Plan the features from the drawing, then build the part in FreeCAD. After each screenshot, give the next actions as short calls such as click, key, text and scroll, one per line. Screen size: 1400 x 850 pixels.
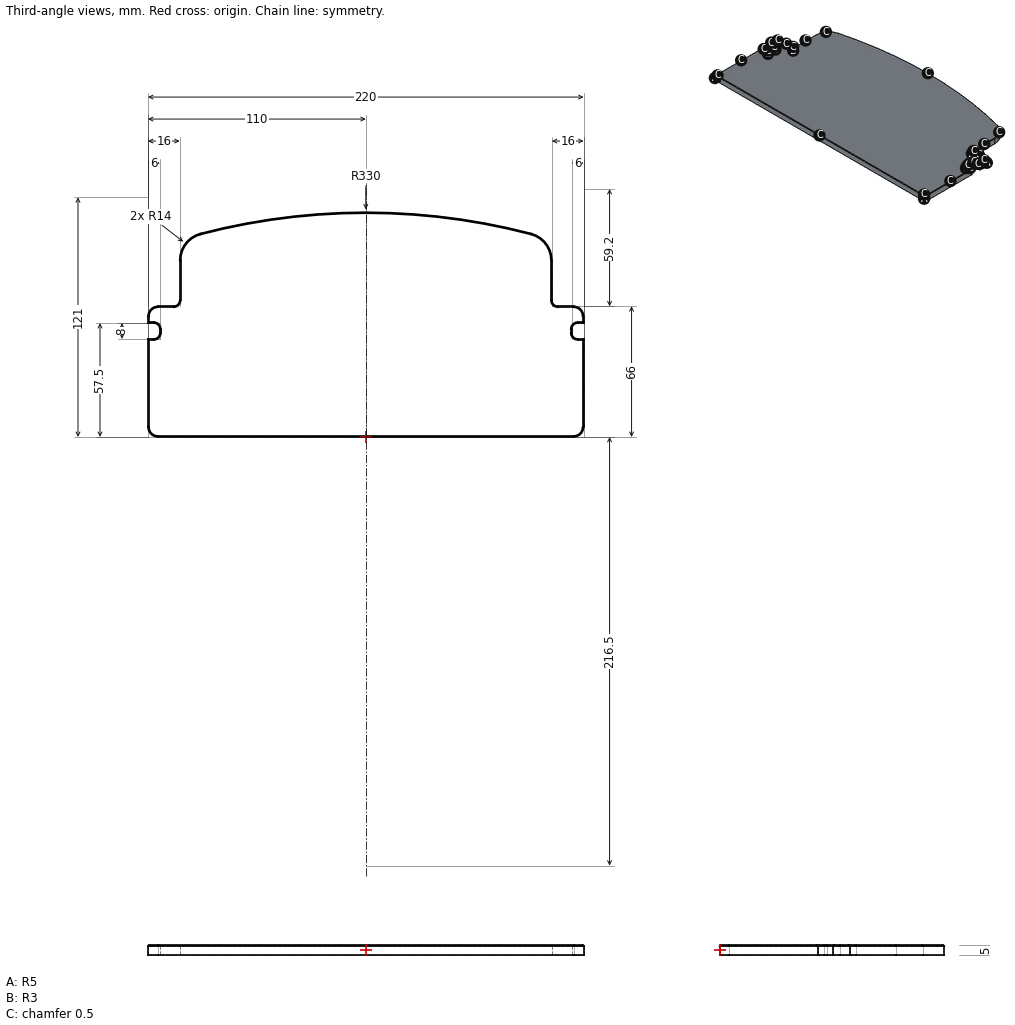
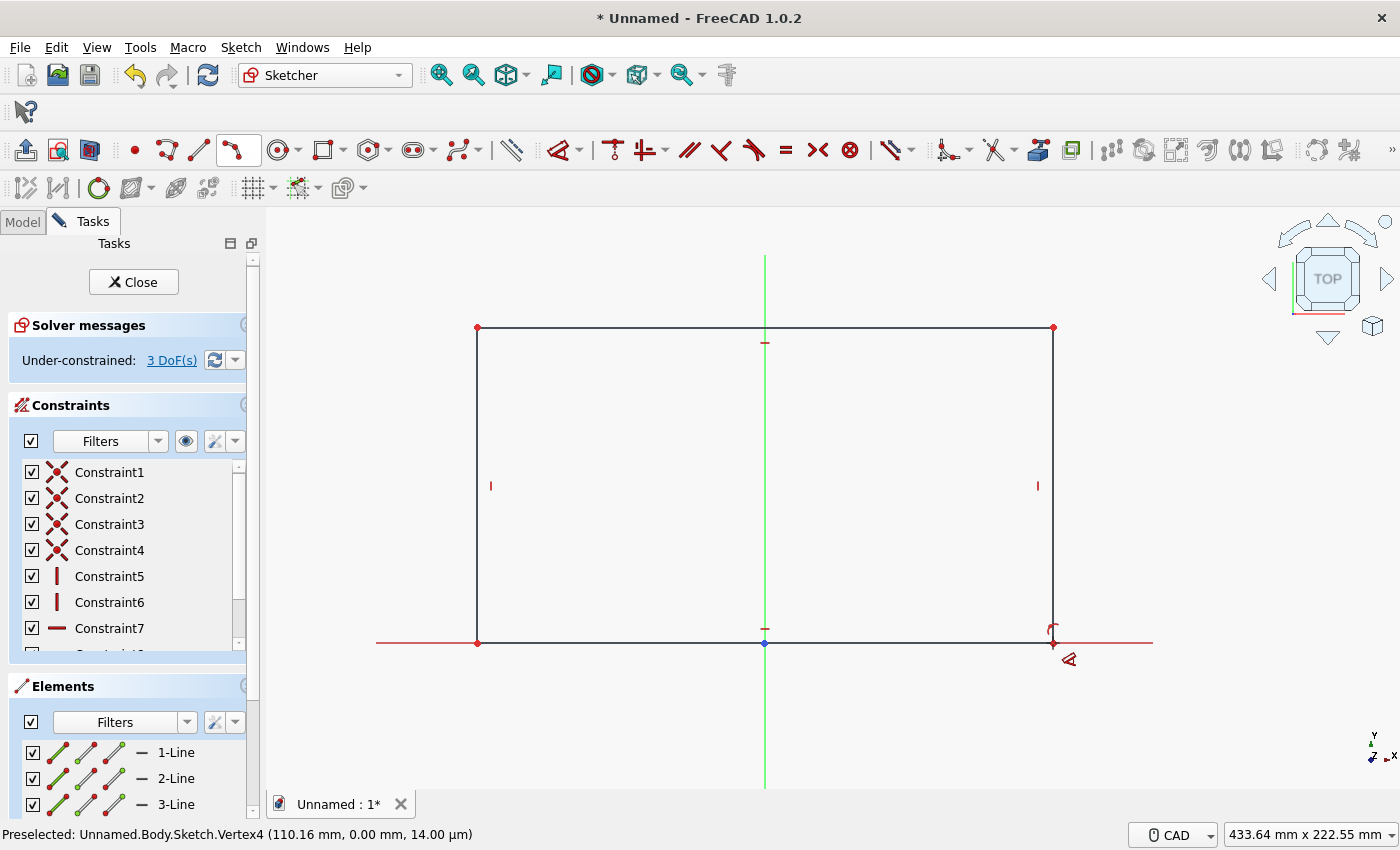
click(477, 423)
click(443, 486)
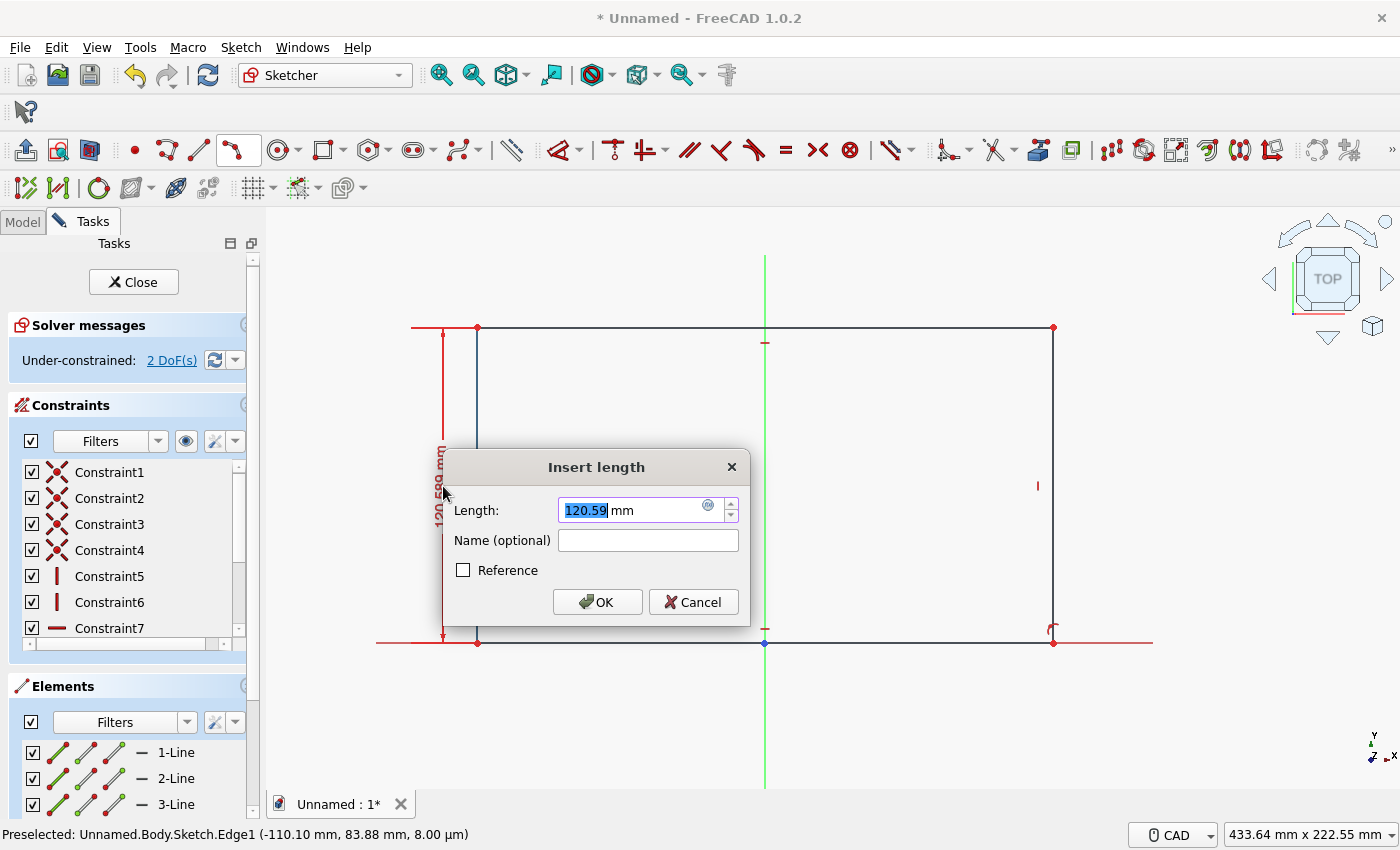
text(121)
key(Return)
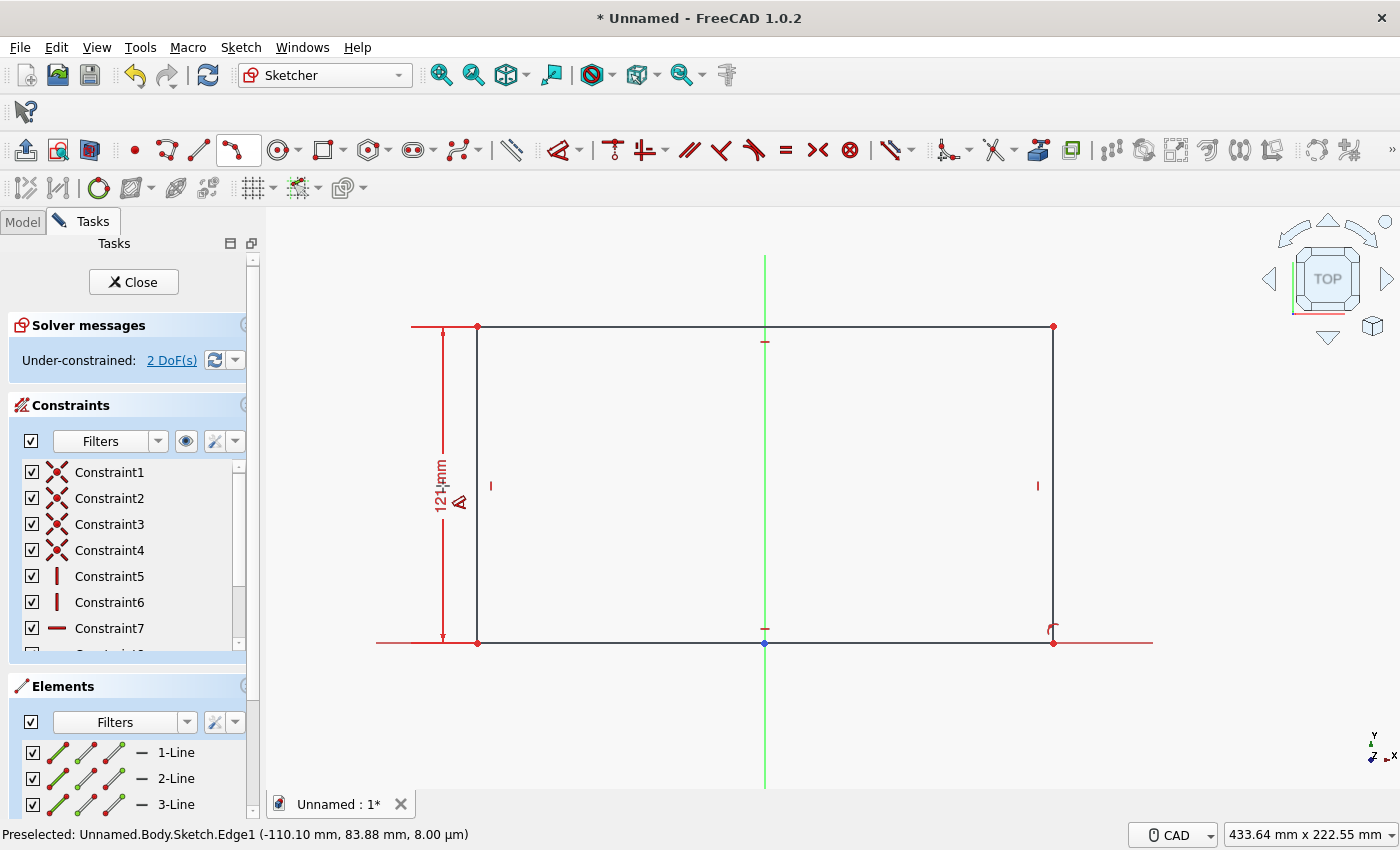
click(650, 643)
click(633, 677)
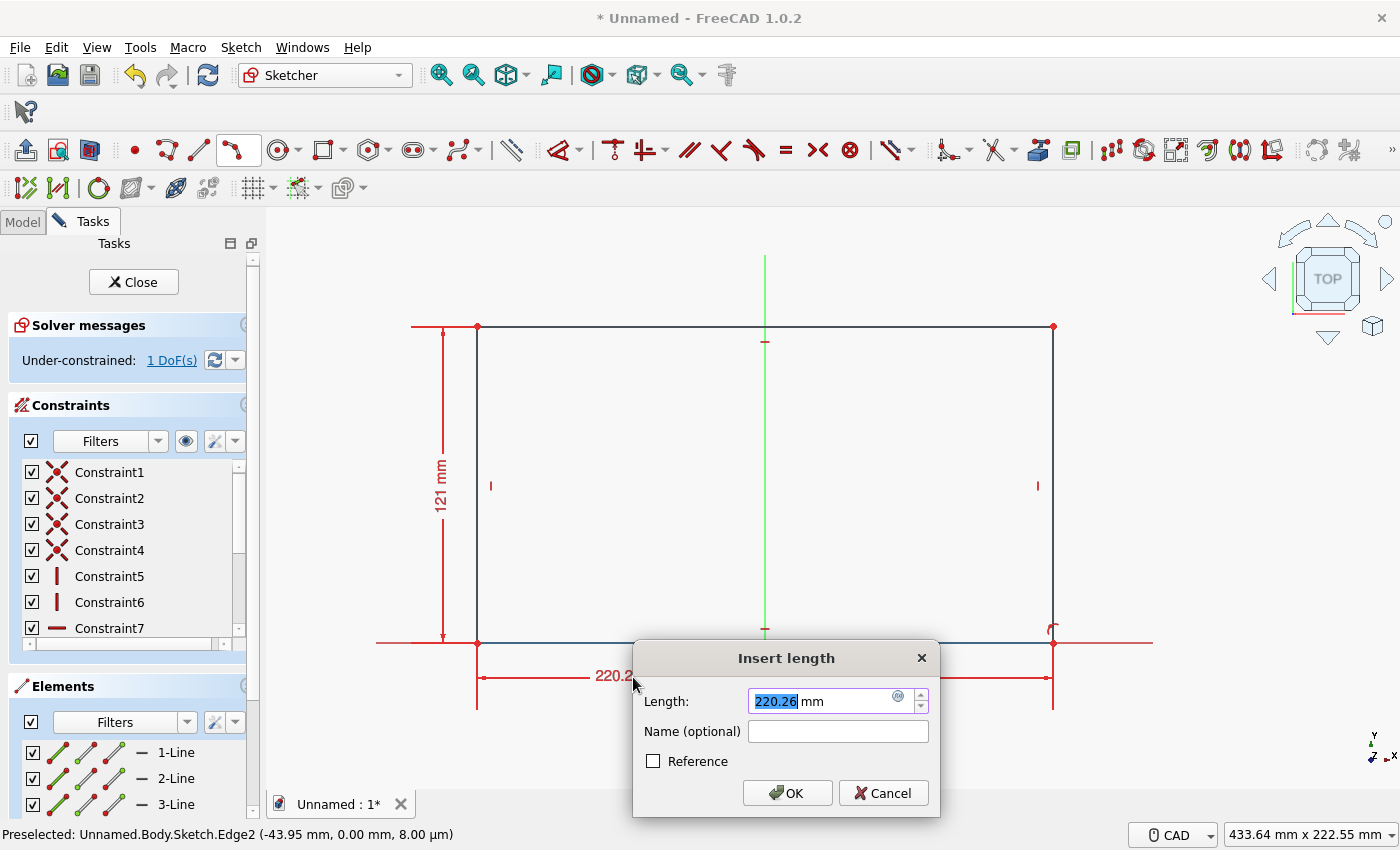
text(220)
key(Return)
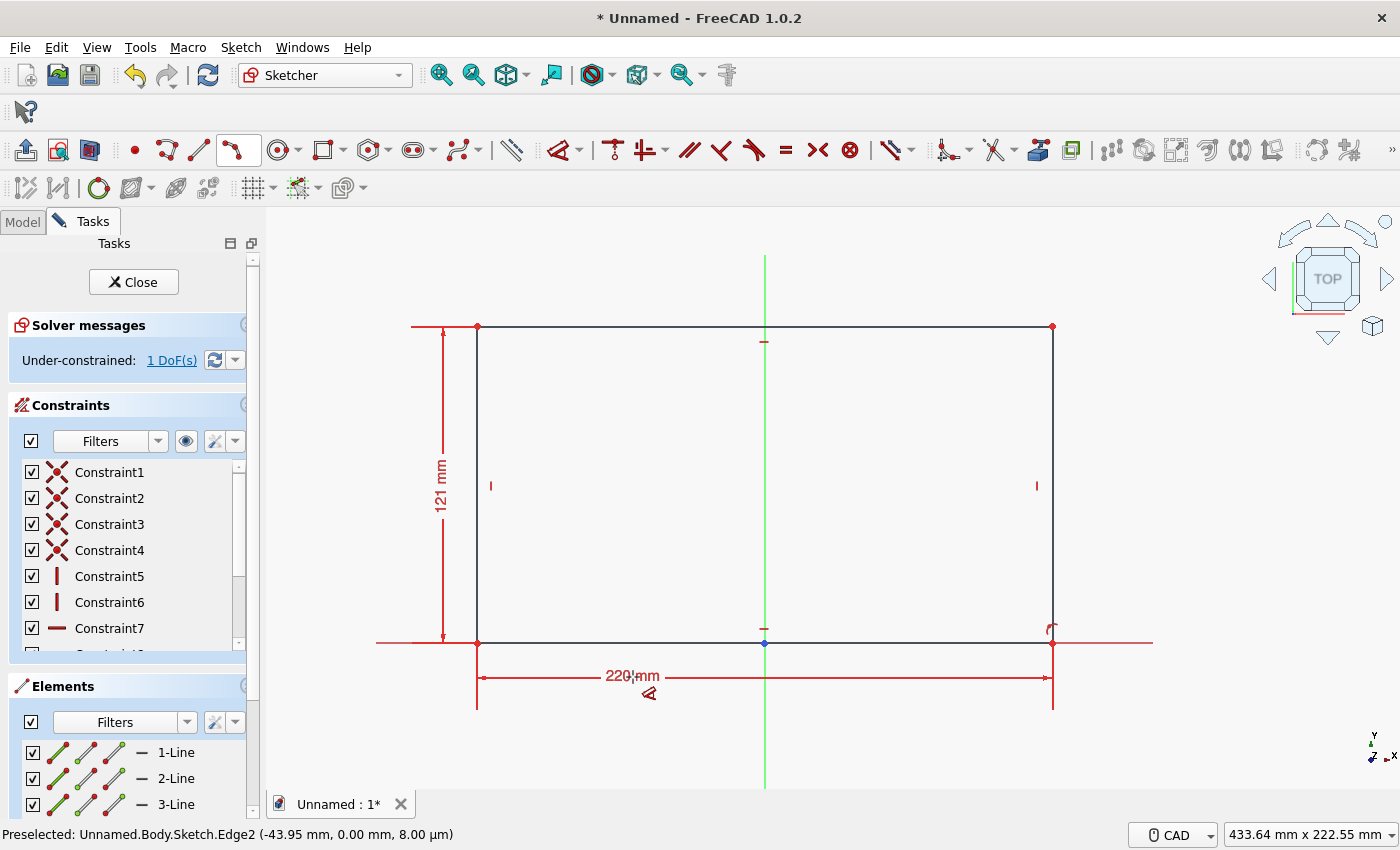
click(477, 327)
click(555, 677)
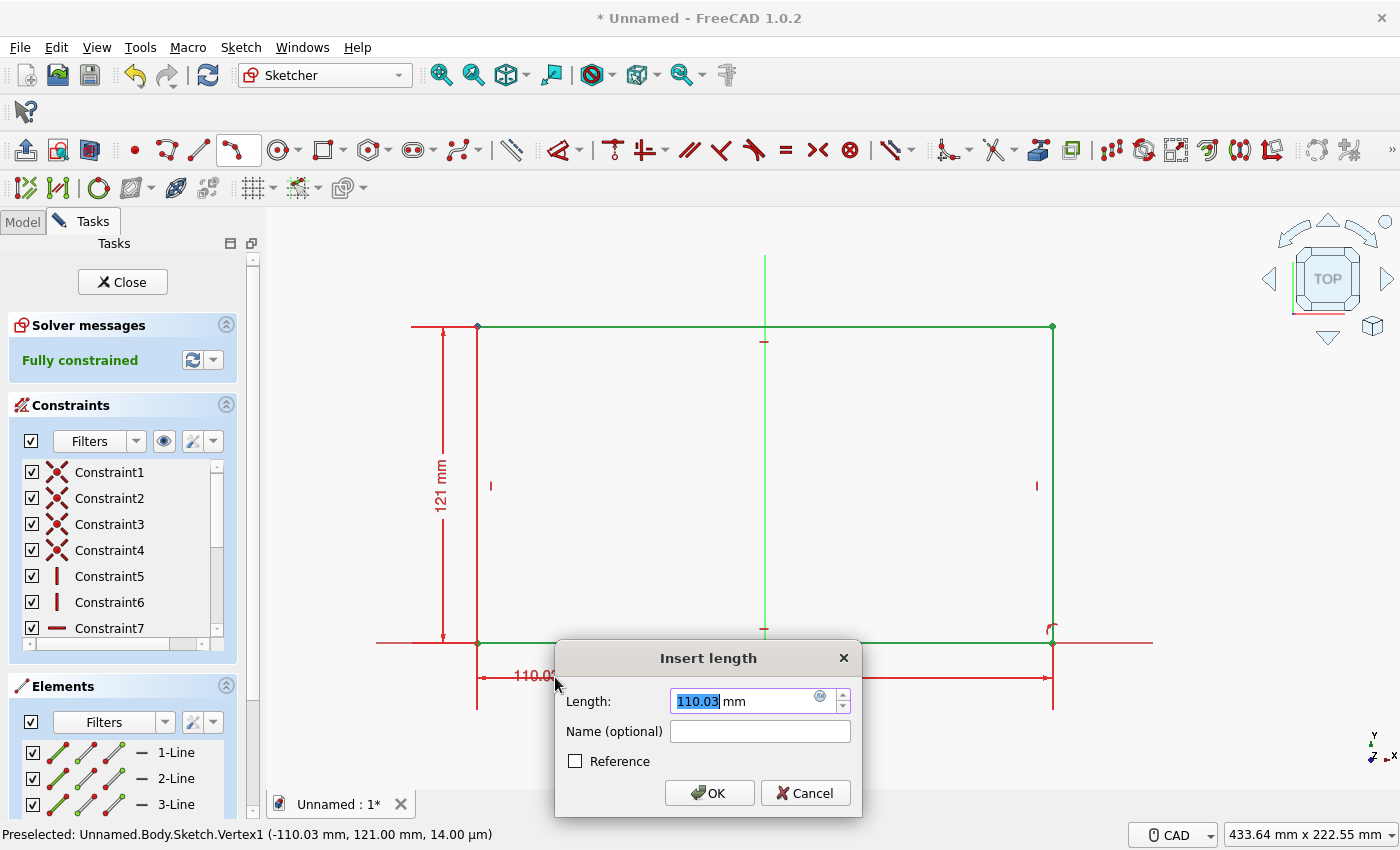
text(110)
key(Return)
key(Escape)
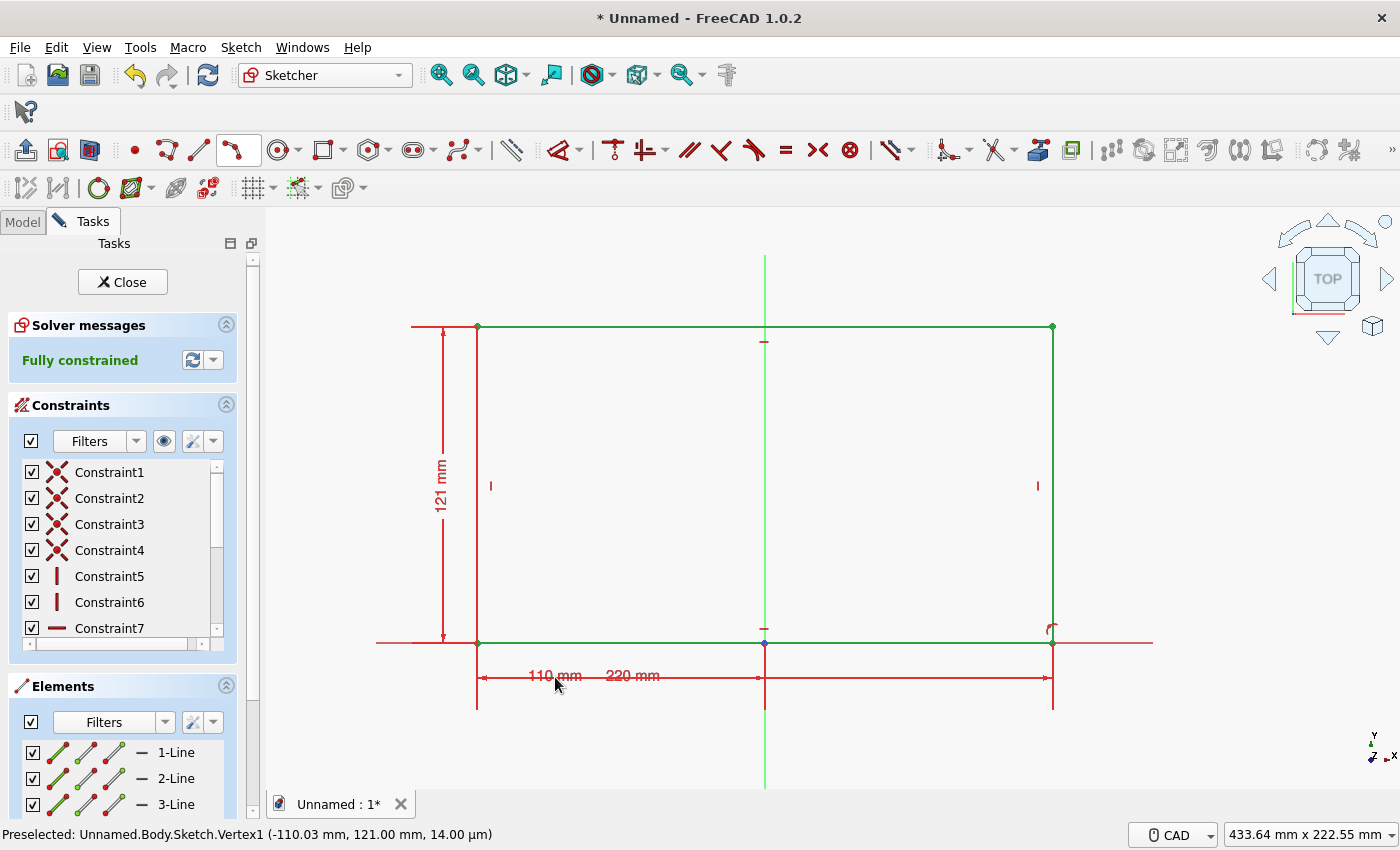
click(123, 282)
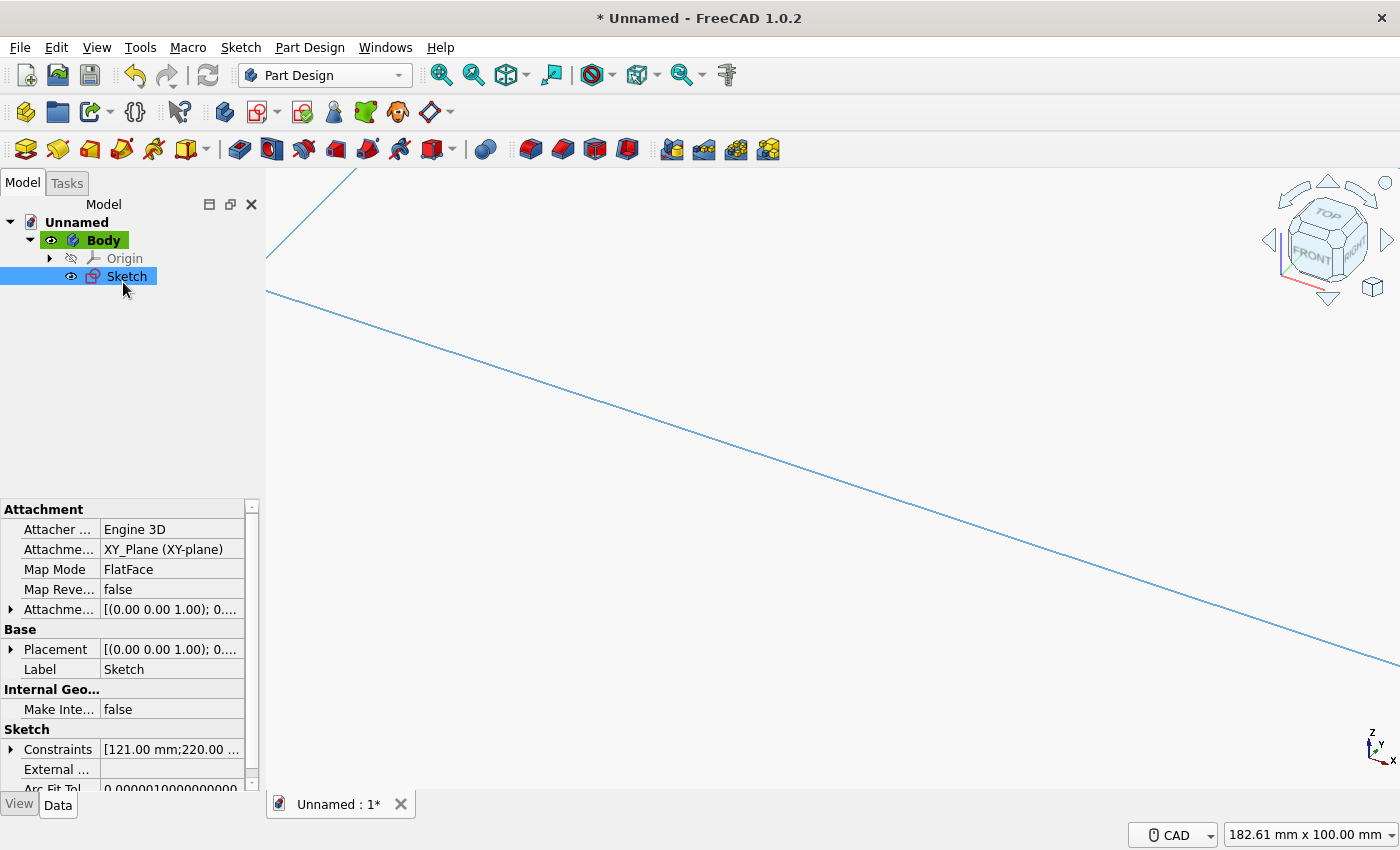
click(26, 150)